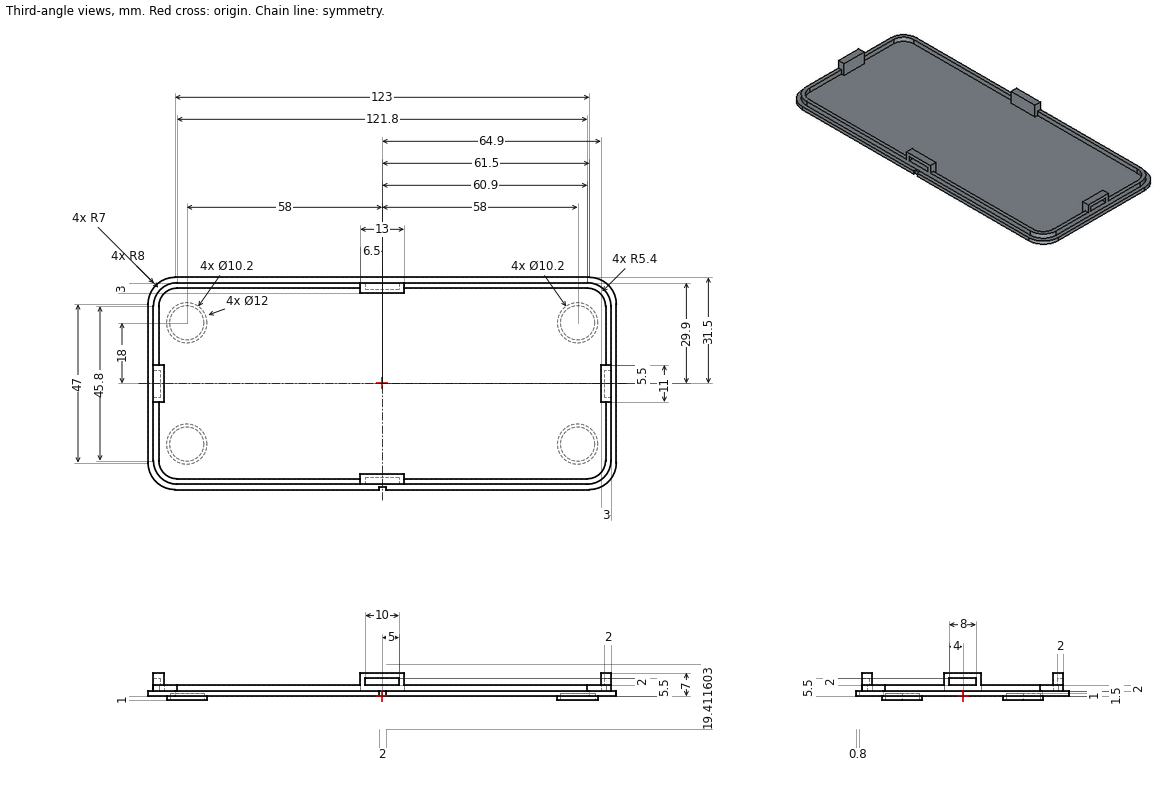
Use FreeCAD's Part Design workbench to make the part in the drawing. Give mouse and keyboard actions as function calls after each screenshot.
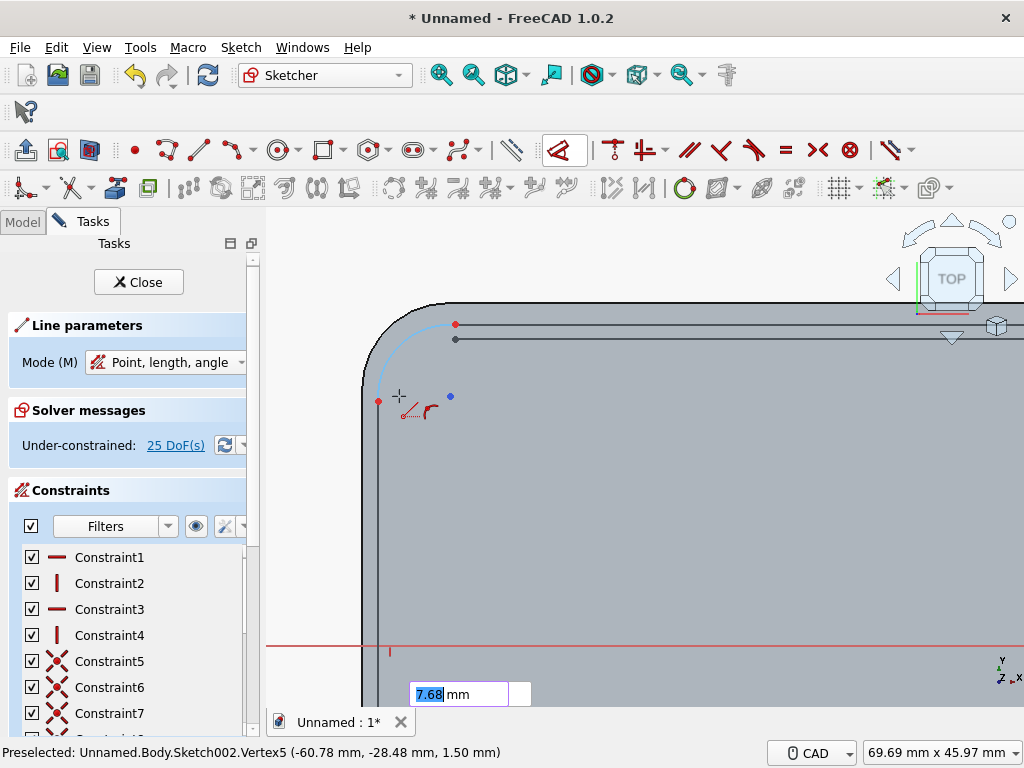
click(397, 397)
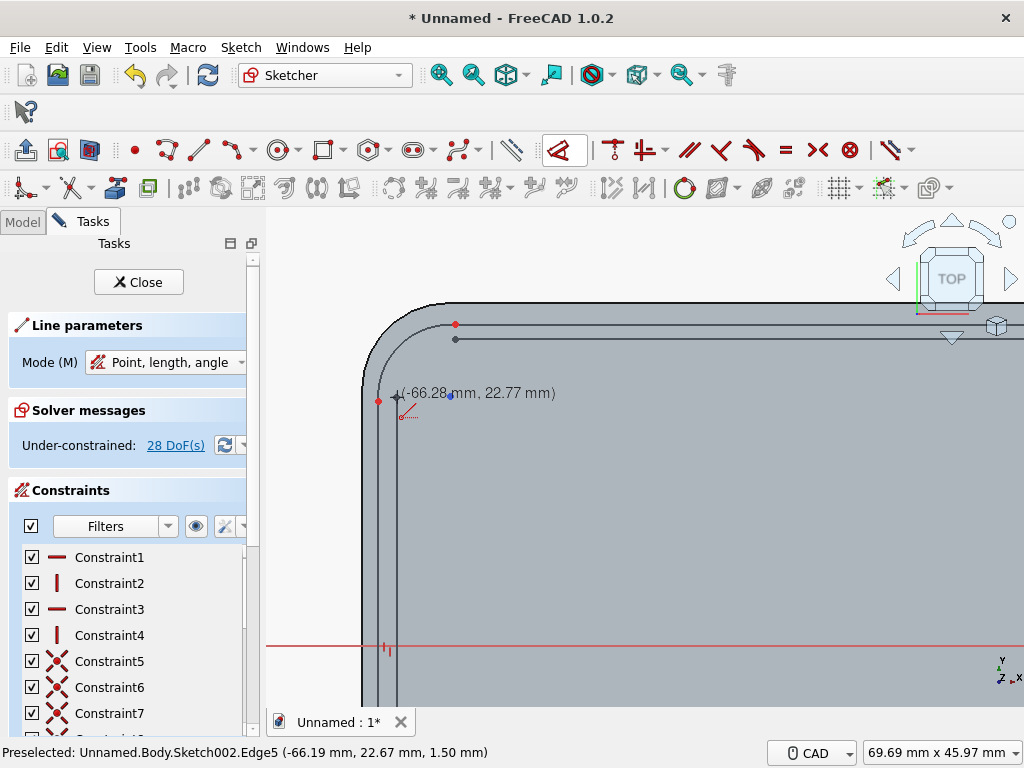
key(g)
key(3)
key(a)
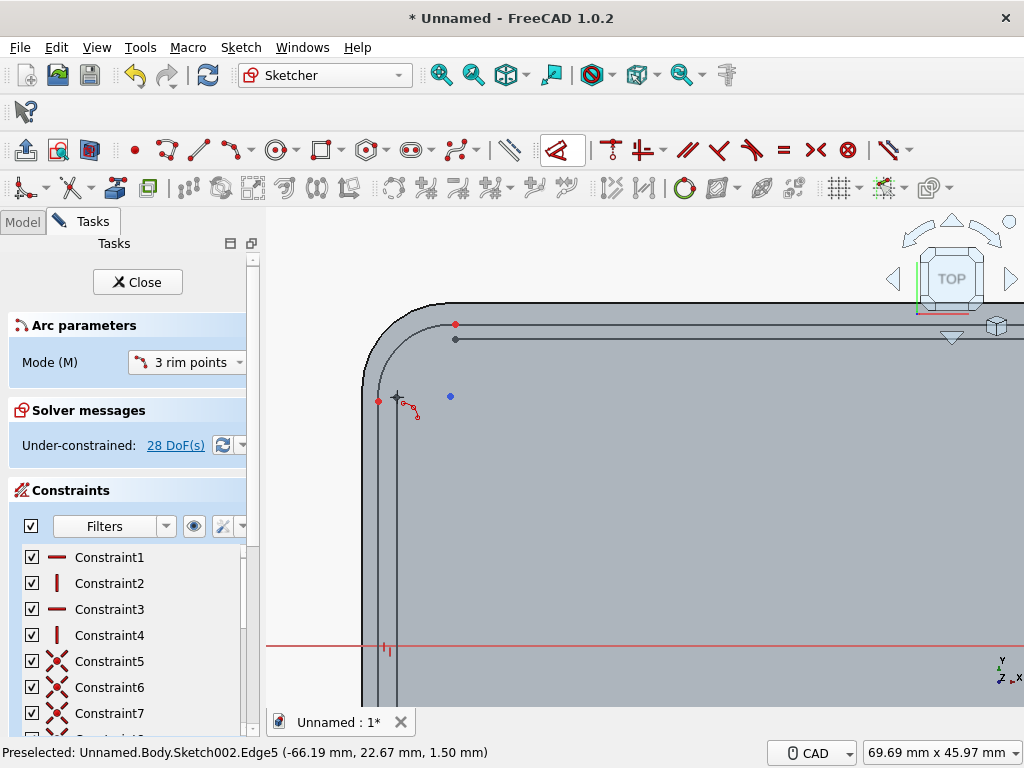
scroll(399, 395, down, 7)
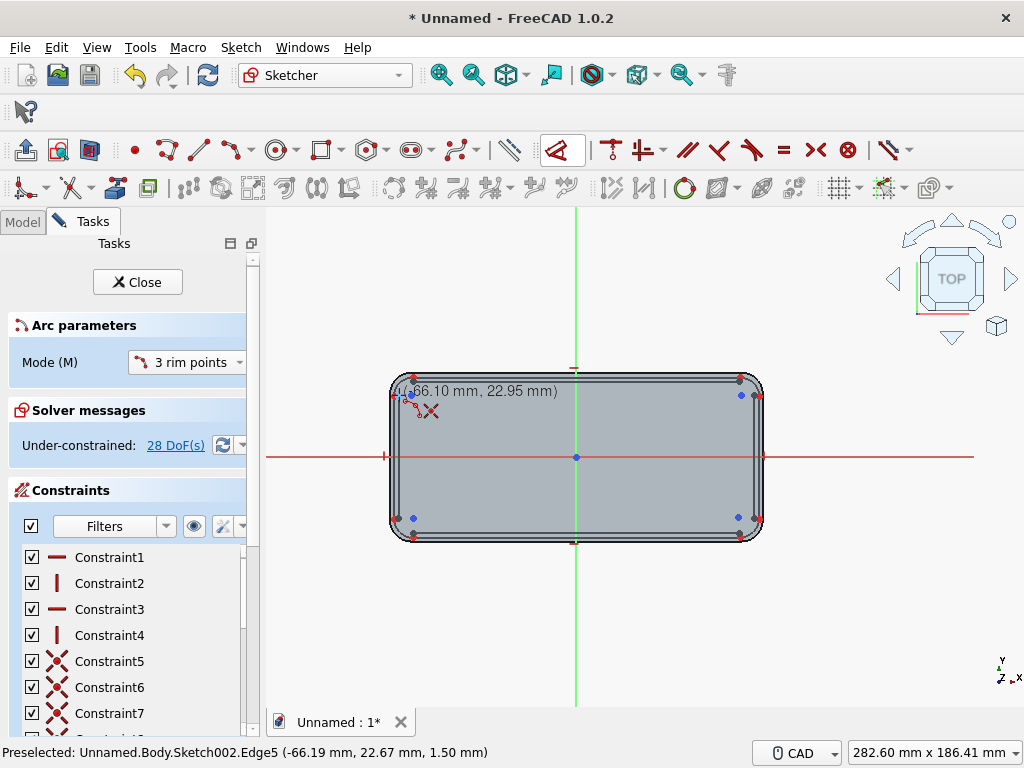
scroll(740, 381, up, 7)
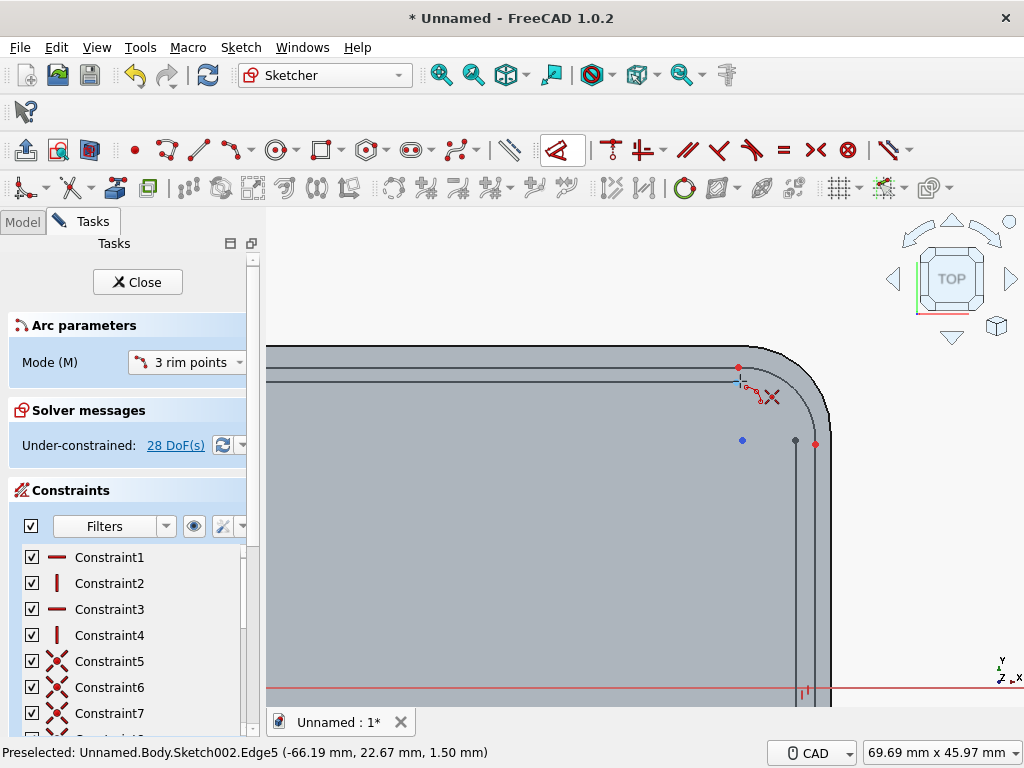
click(737, 382)
click(796, 440)
click(779, 398)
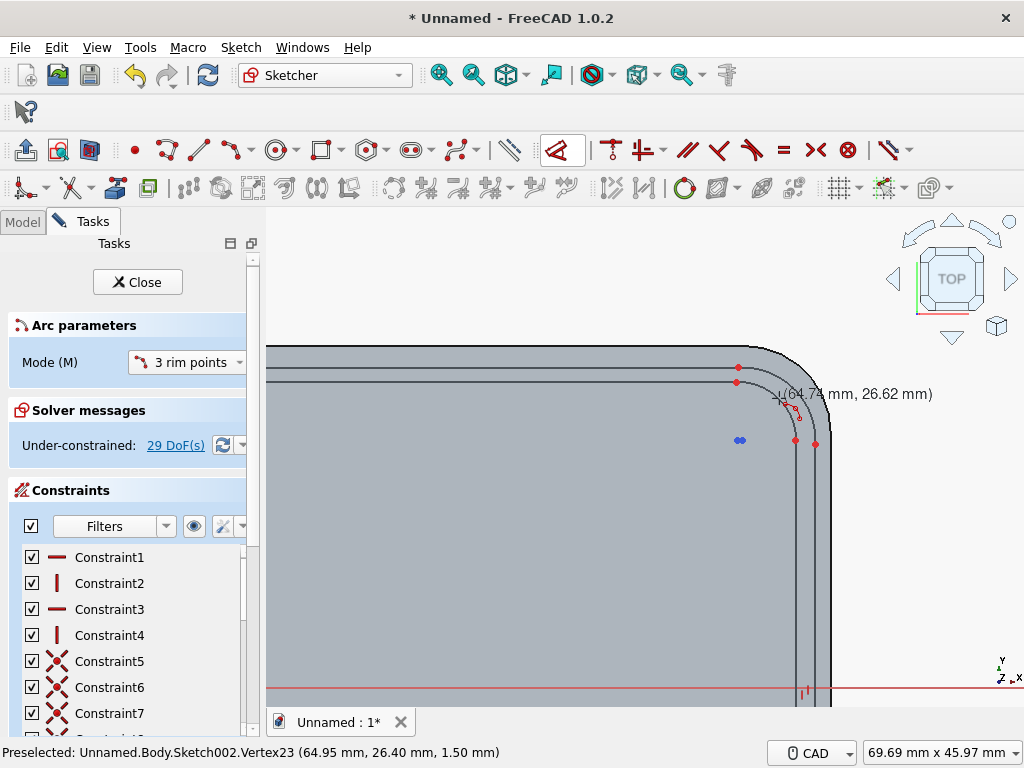
scroll(741, 381, down, 7)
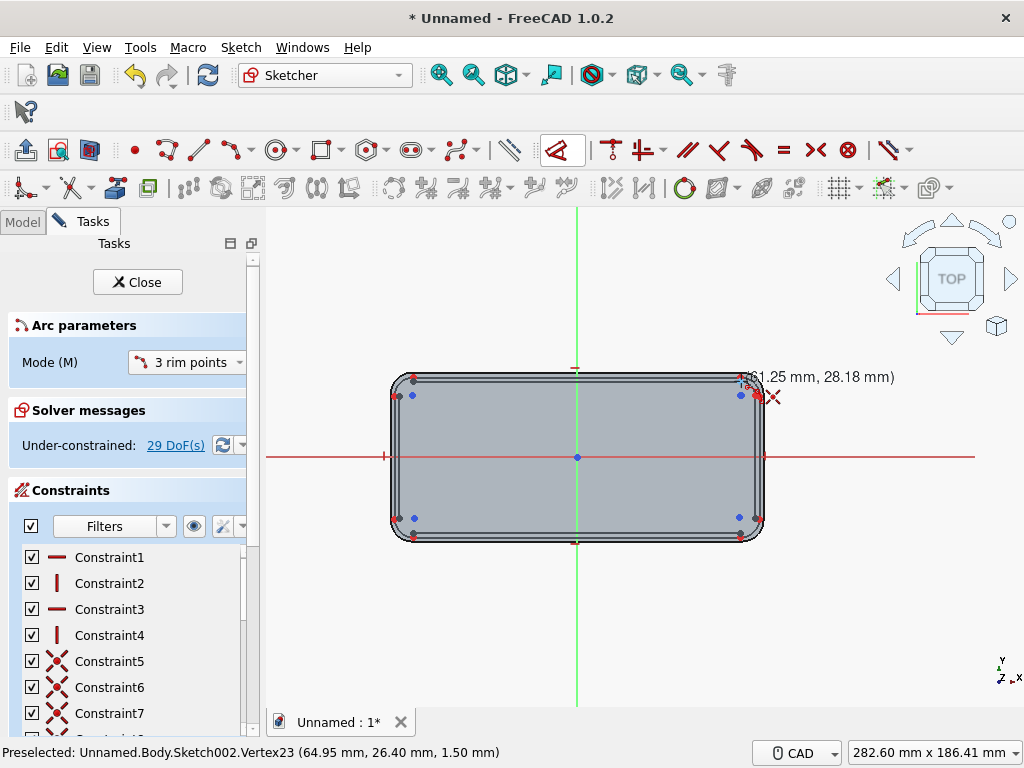
scroll(755, 519, up, 7)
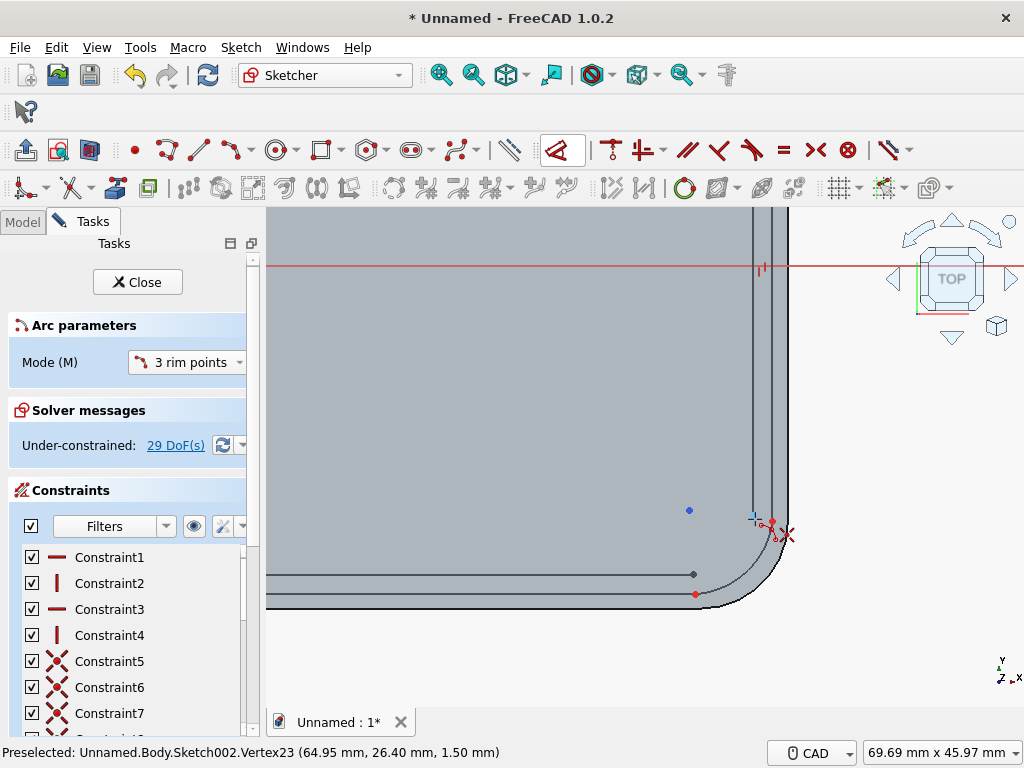
click(753, 516)
click(694, 575)
click(736, 557)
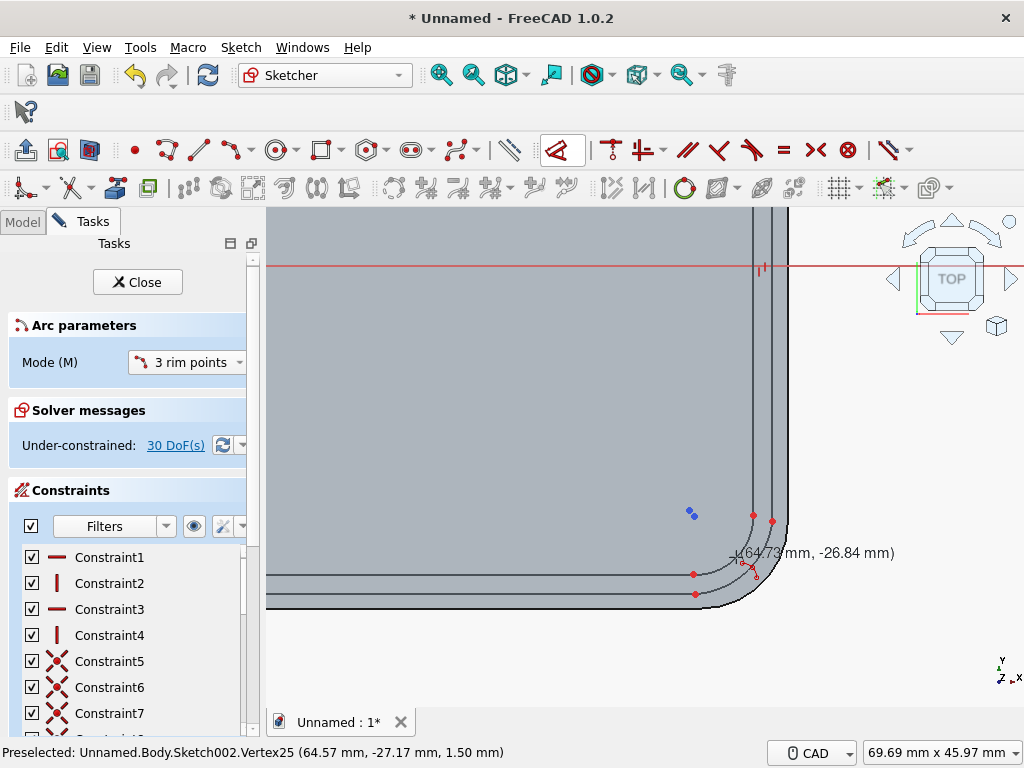
scroll(755, 520, down, 7)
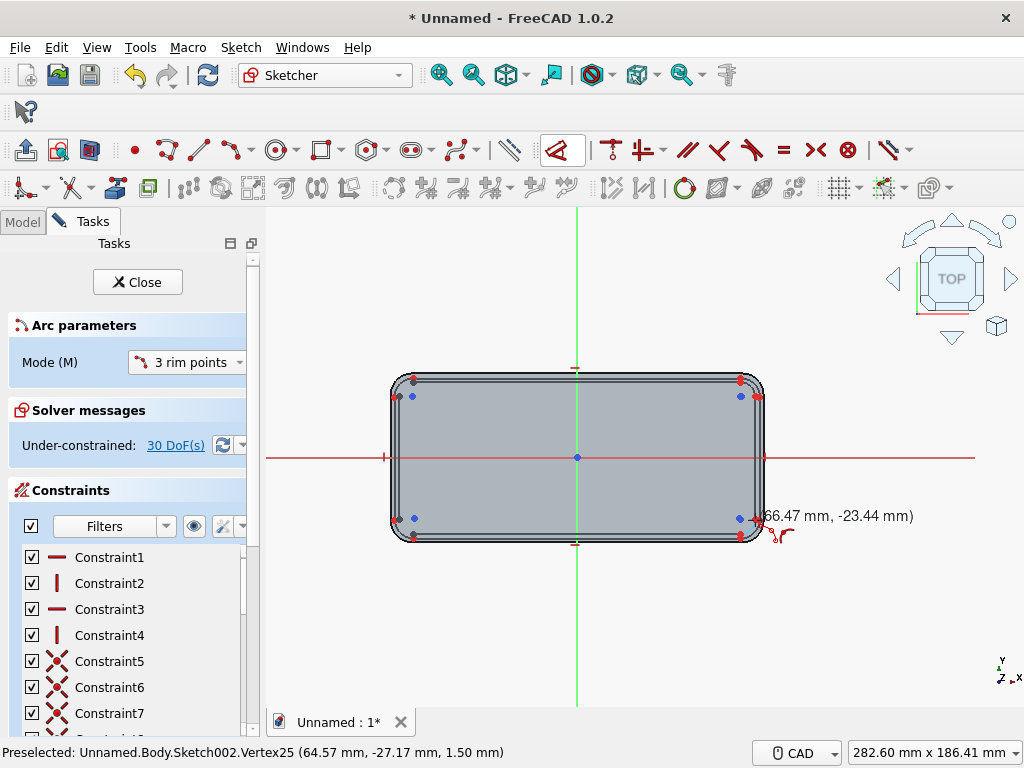
scroll(414, 534, up, 7)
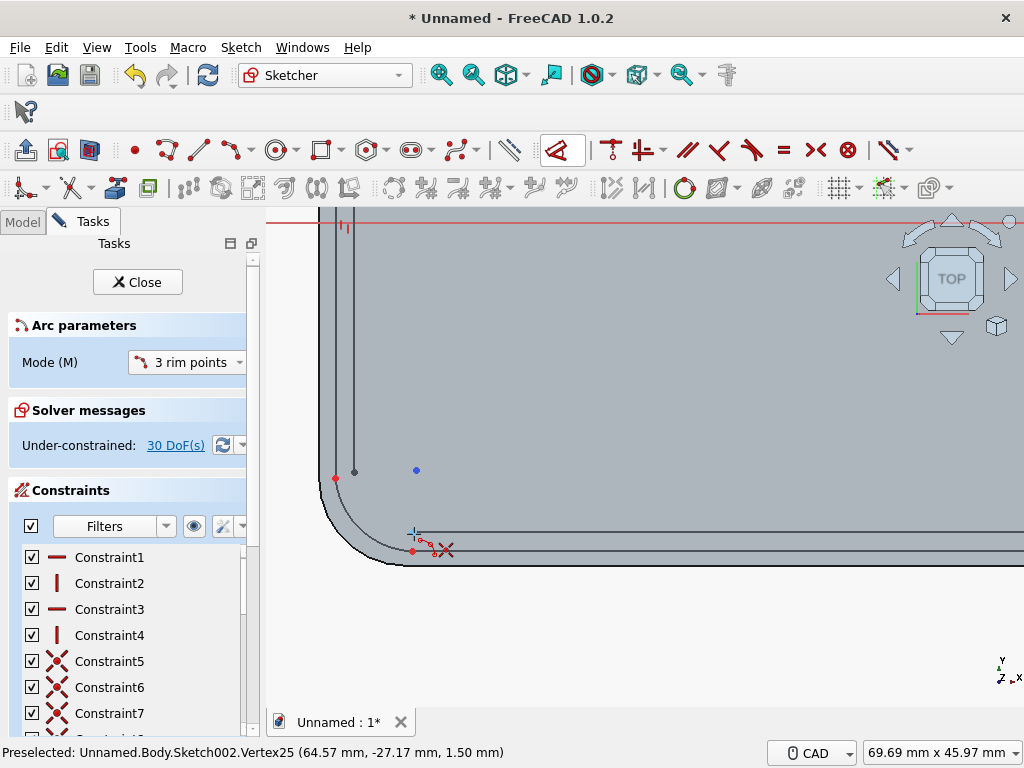
click(413, 532)
click(354, 473)
click(371, 514)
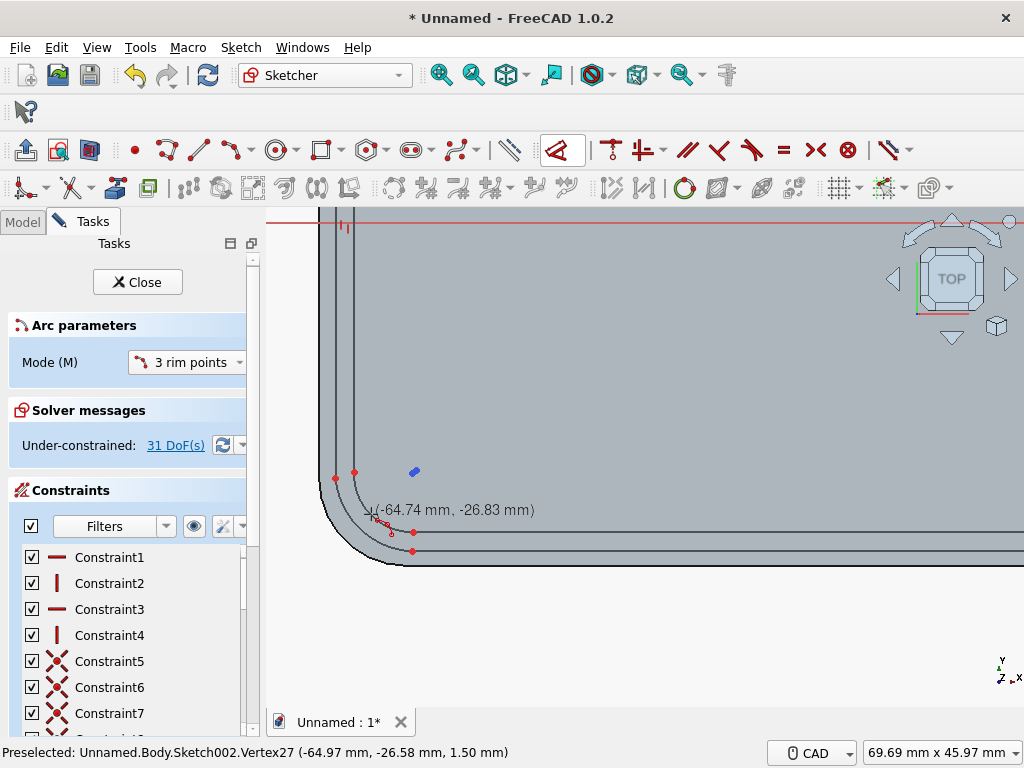
scroll(413, 534, down, 7)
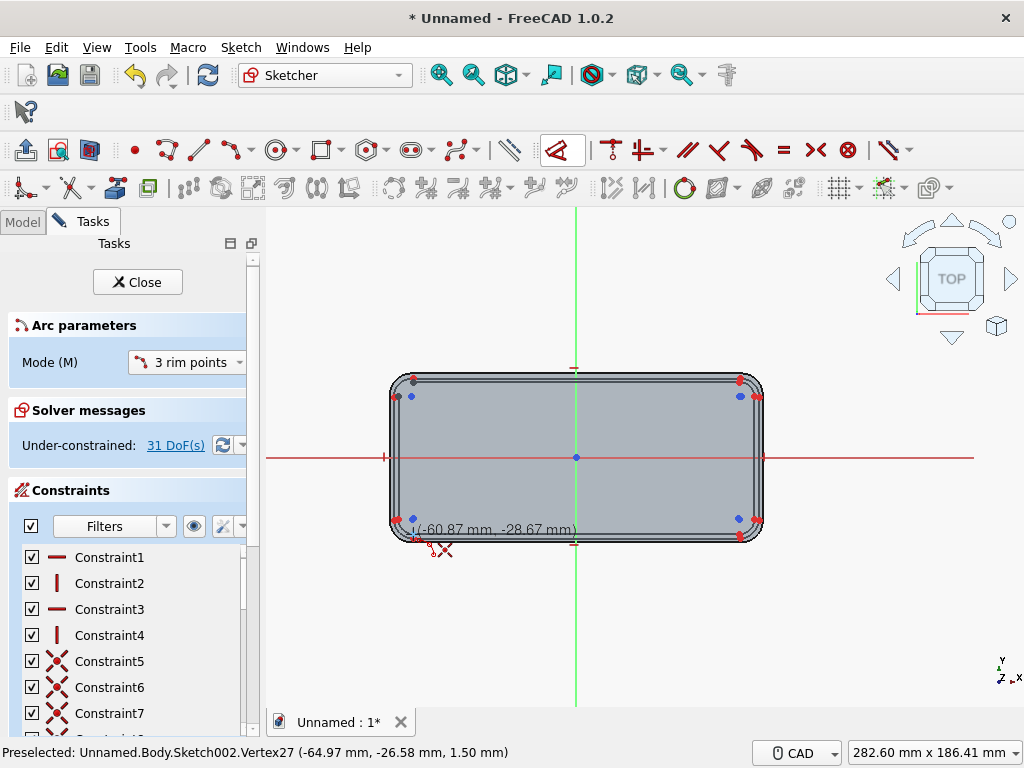
scroll(399, 396, up, 7)